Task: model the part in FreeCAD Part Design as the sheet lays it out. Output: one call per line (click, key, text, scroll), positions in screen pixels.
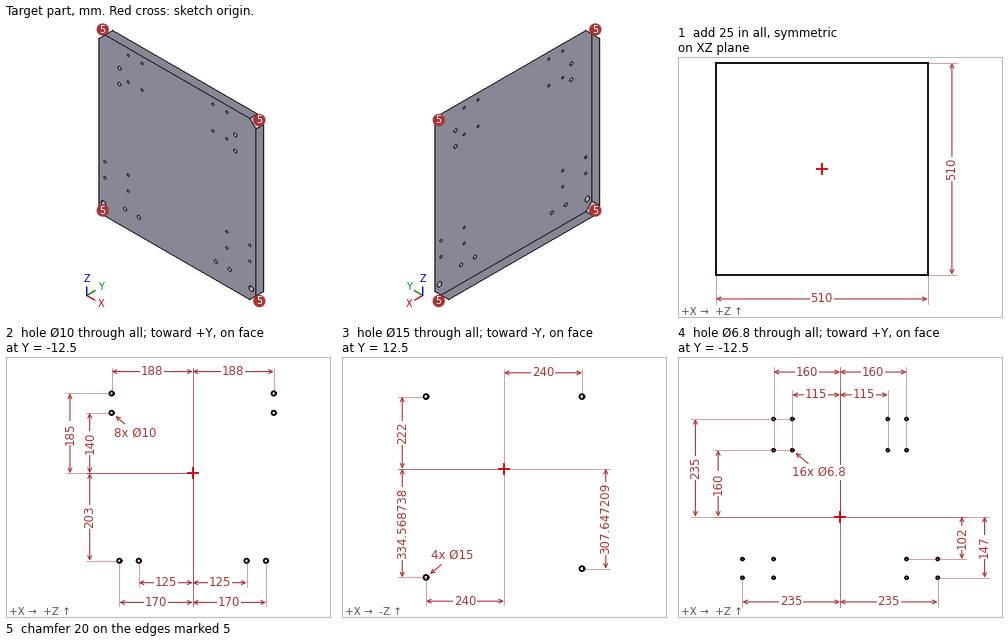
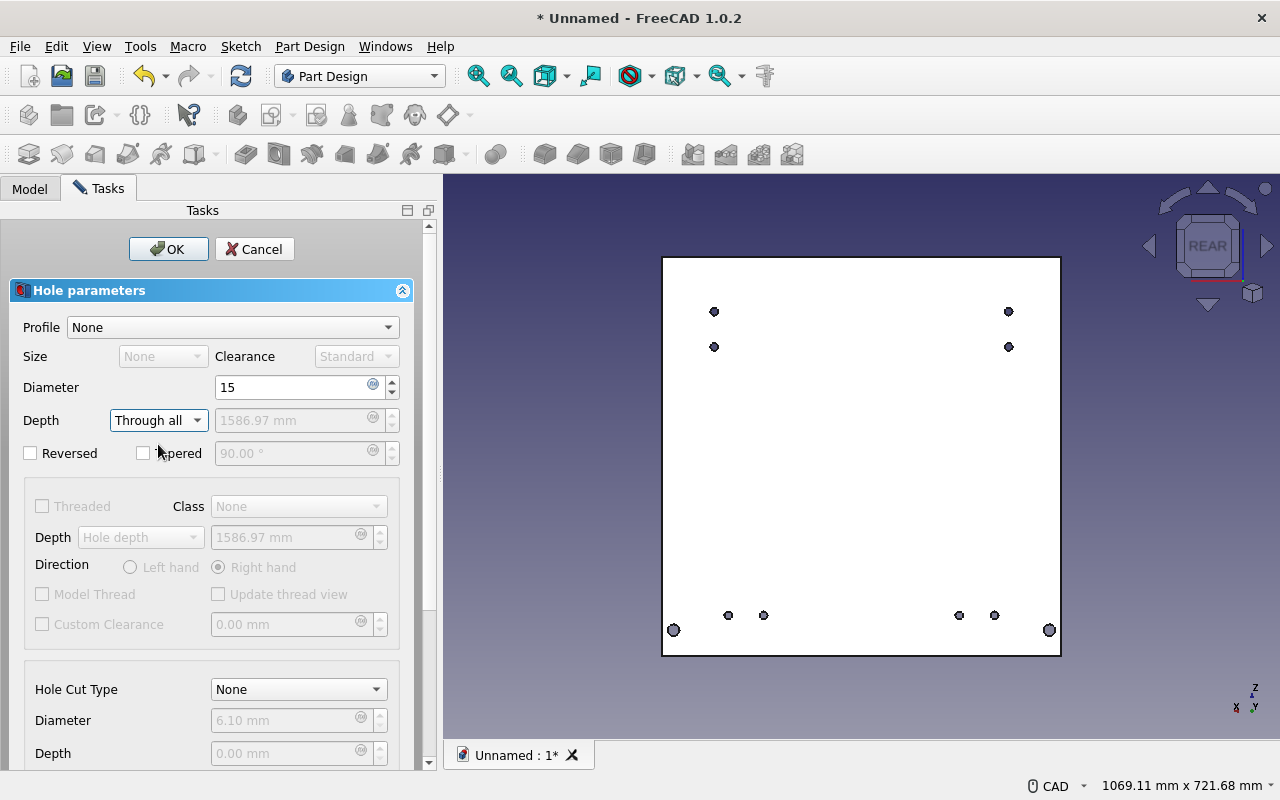
click(169, 249)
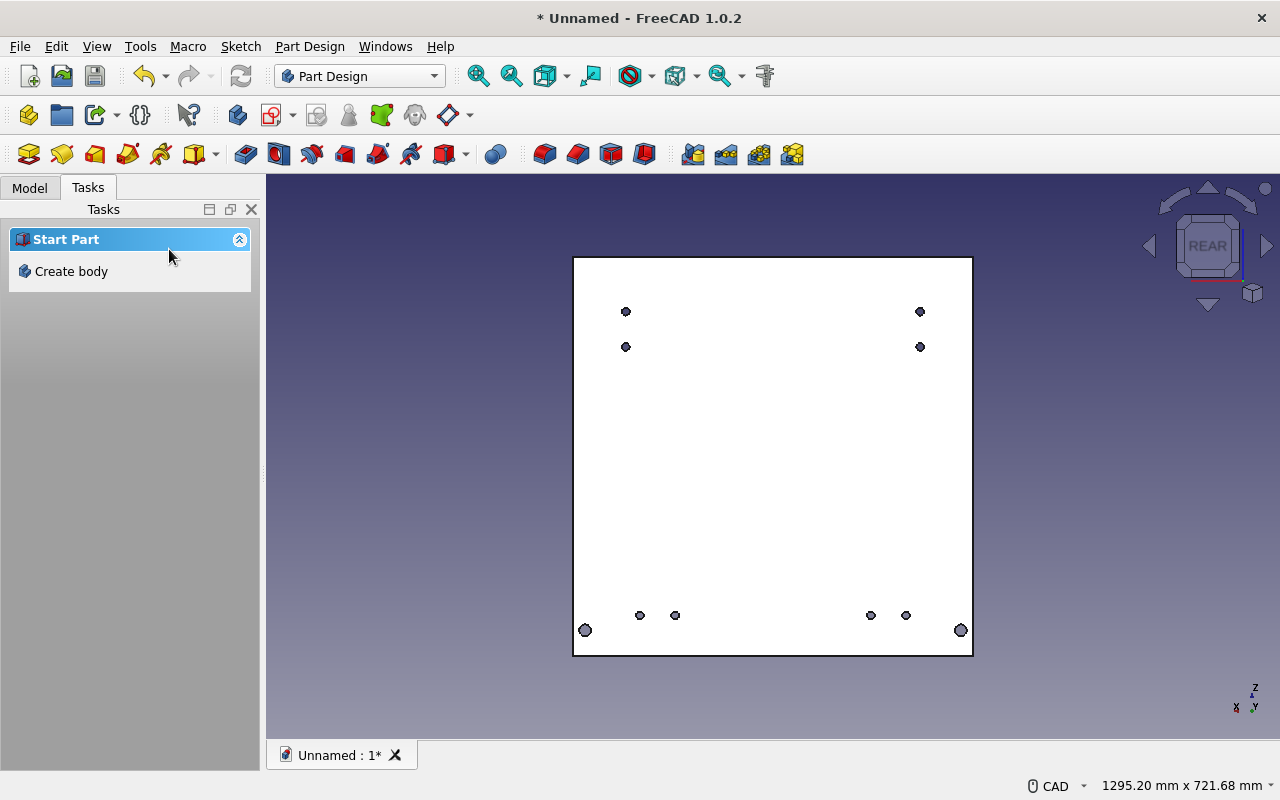
key(0)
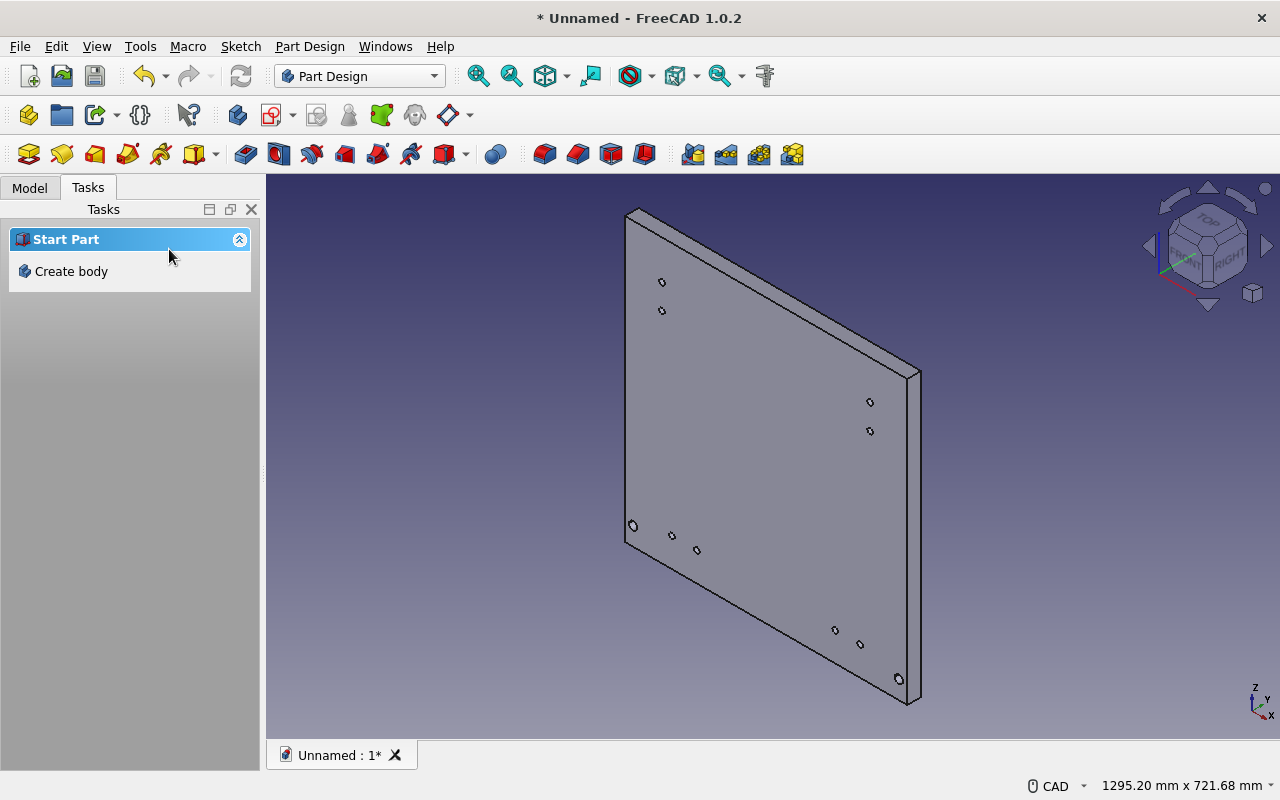
click(766, 459)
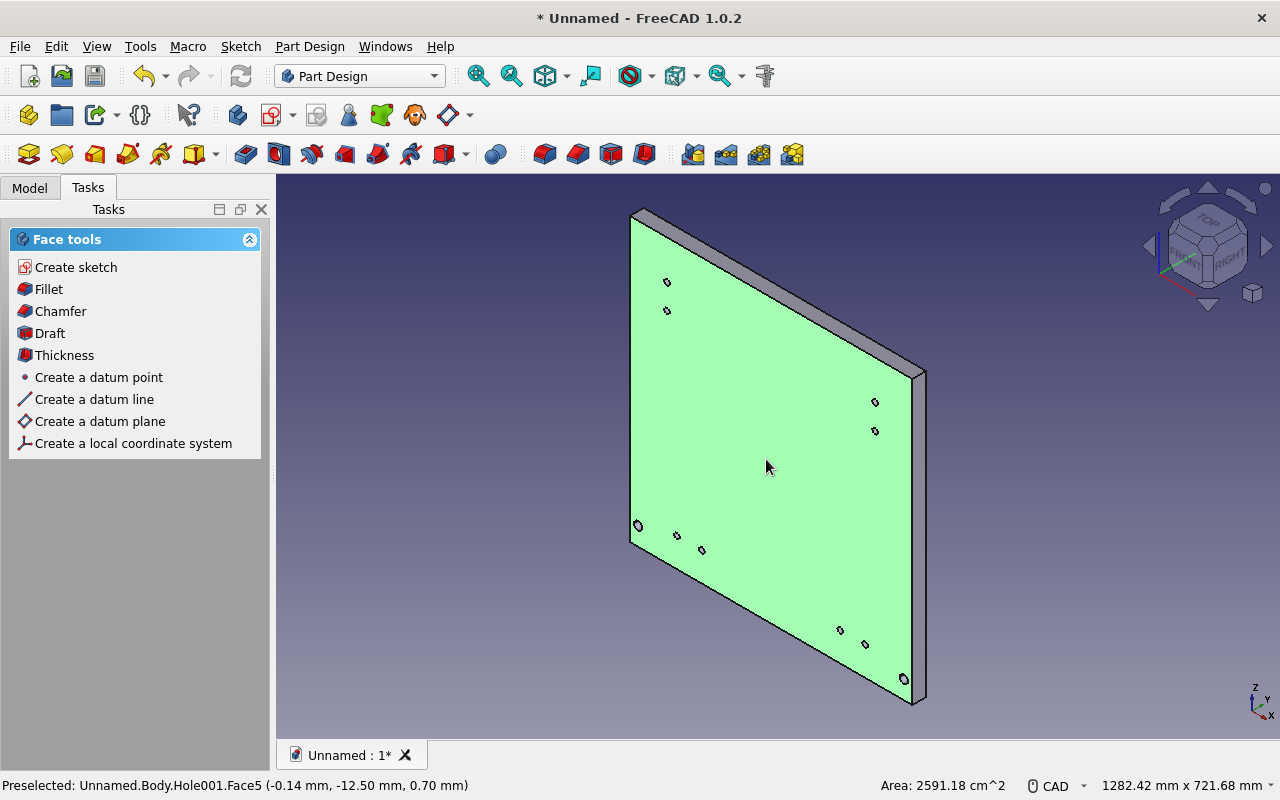
click(270, 116)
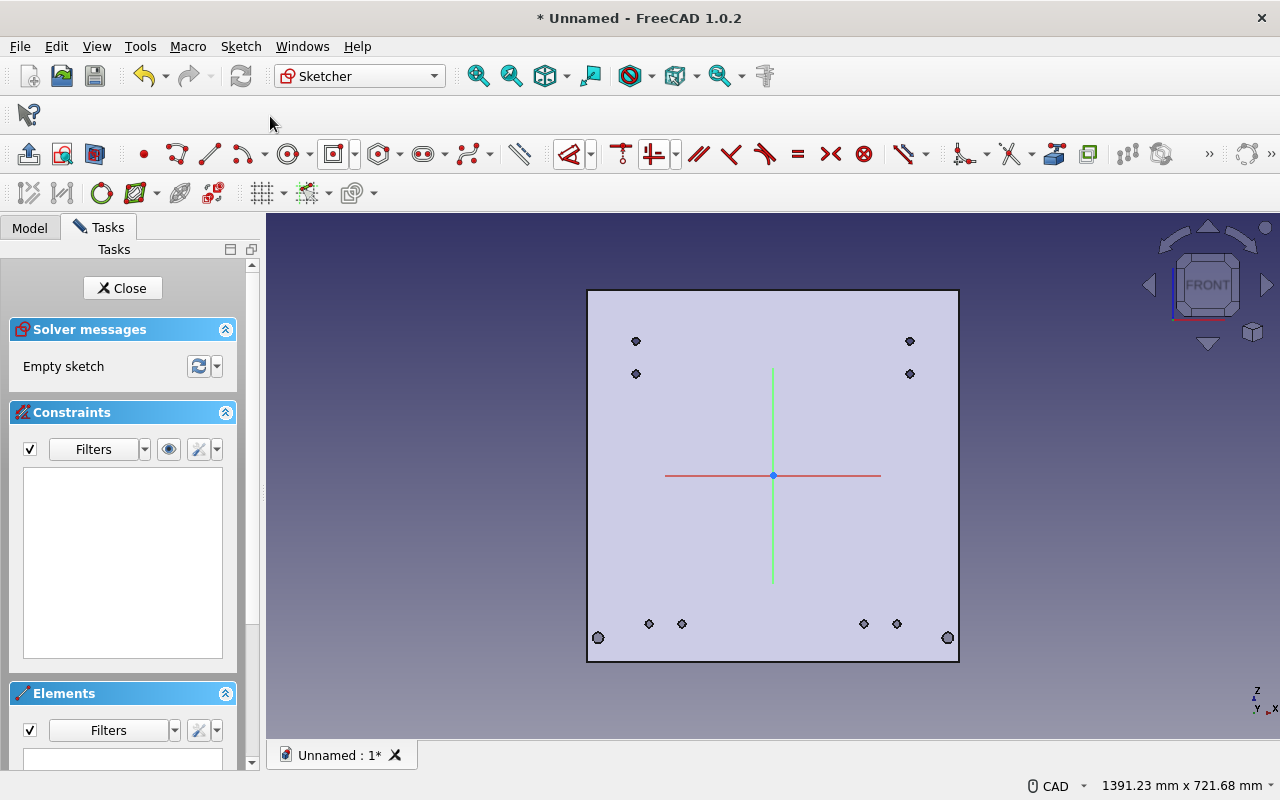
key(g)
key(c)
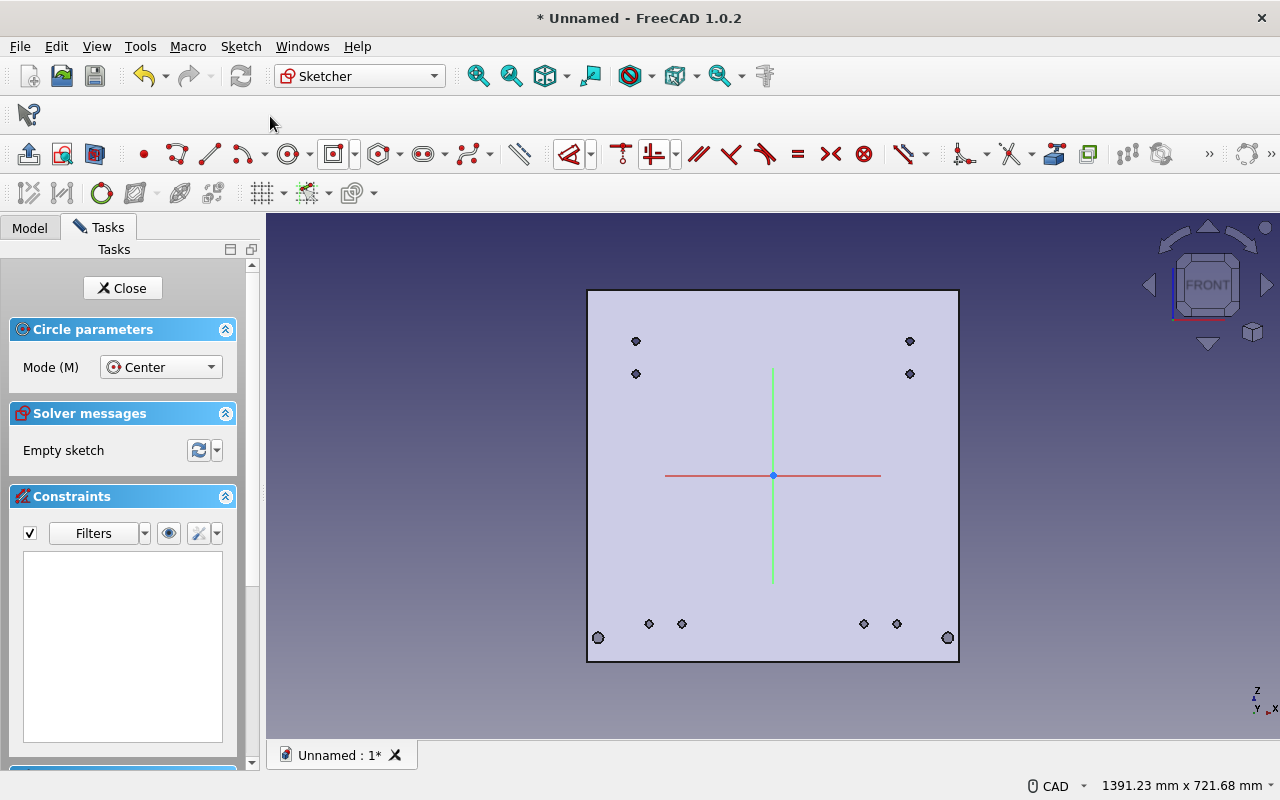
scroll(689, 359, up, 12)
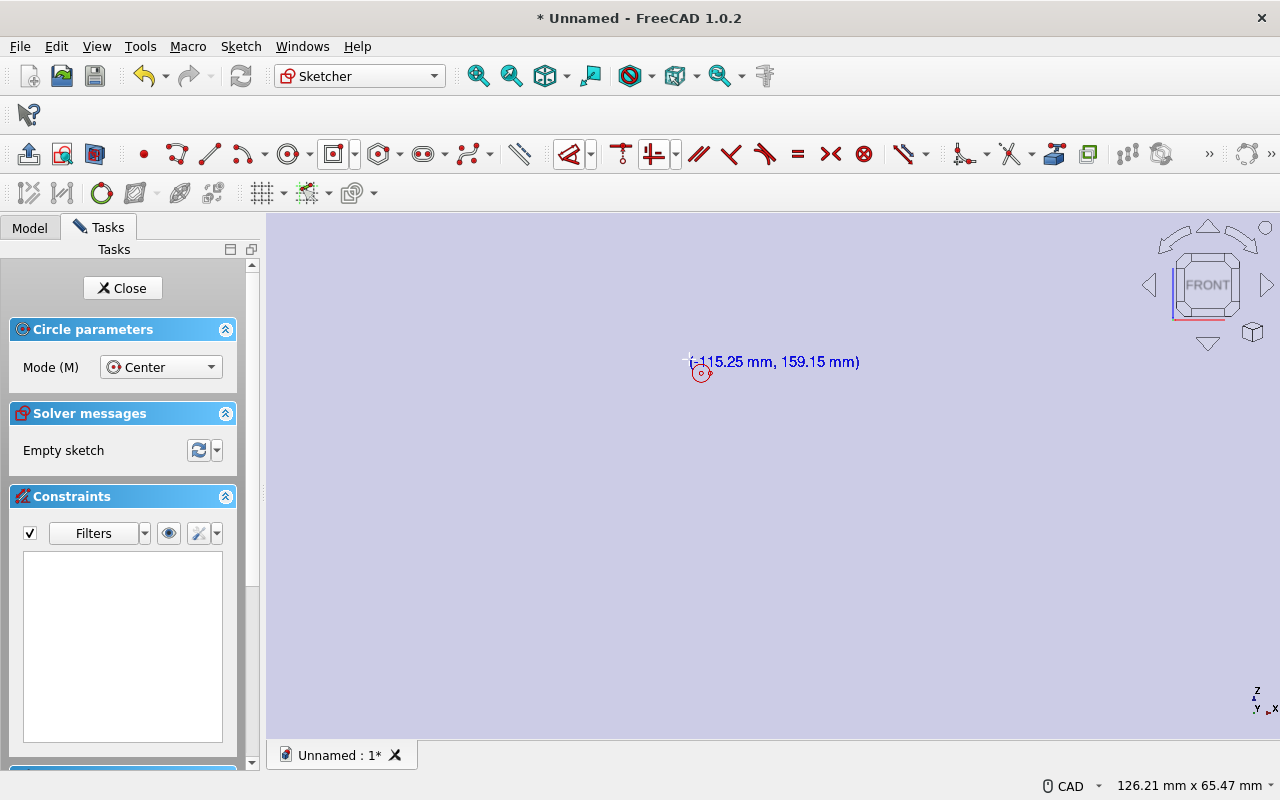
scroll(592, 374, down, 11)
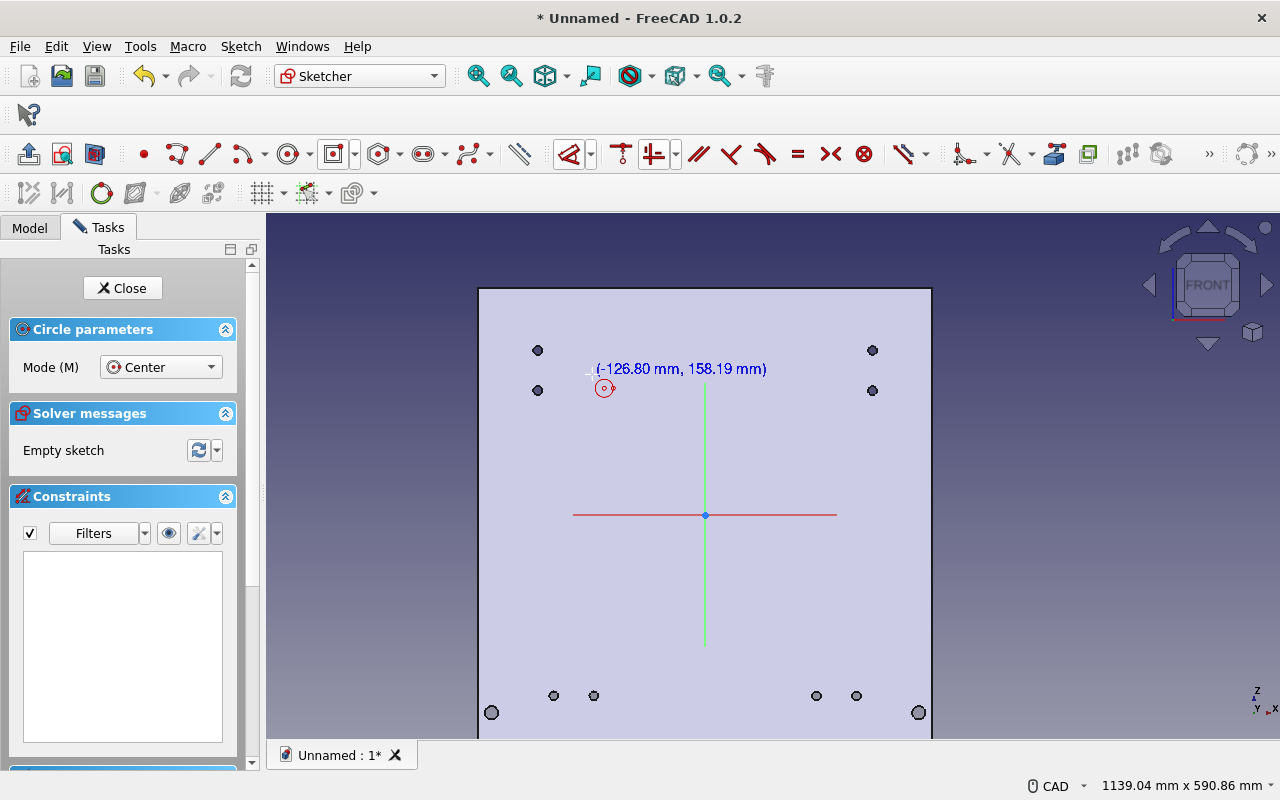
click(603, 373)
move(605, 371)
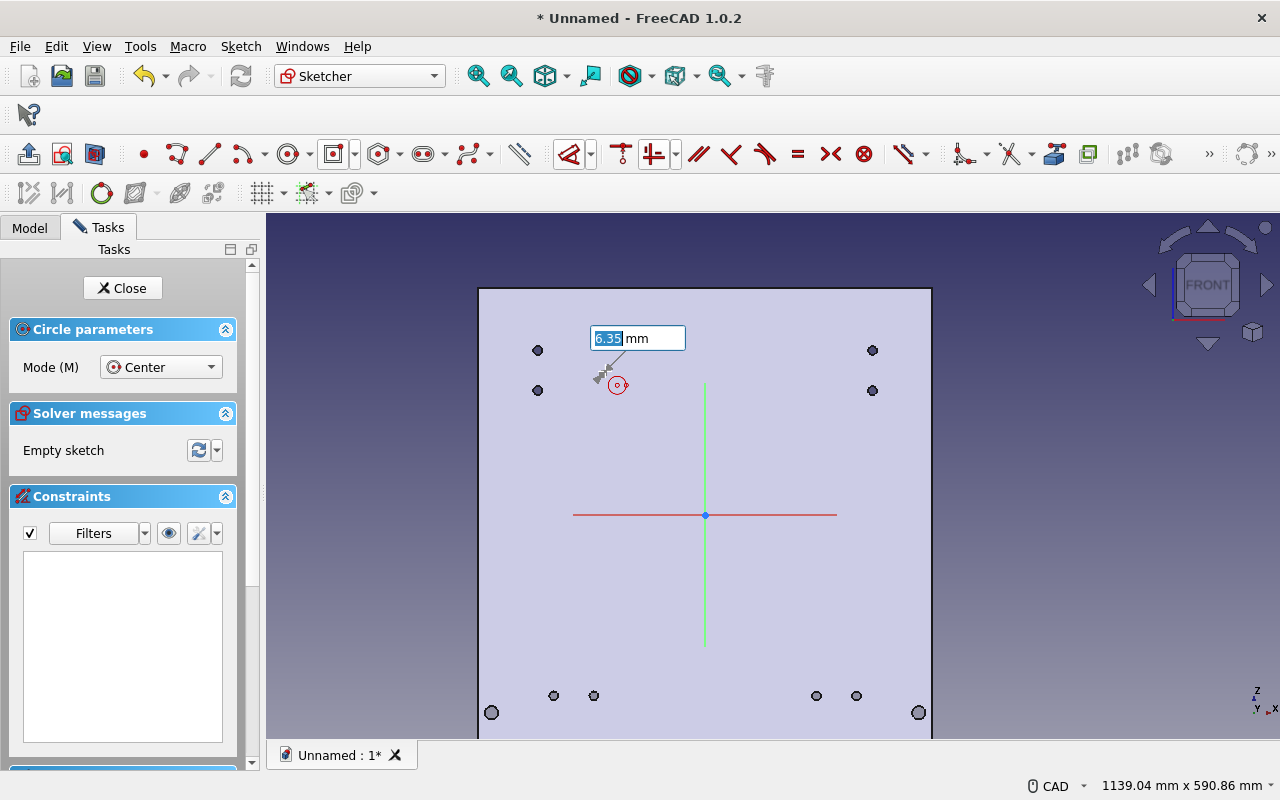
text(6.8)
key(Return)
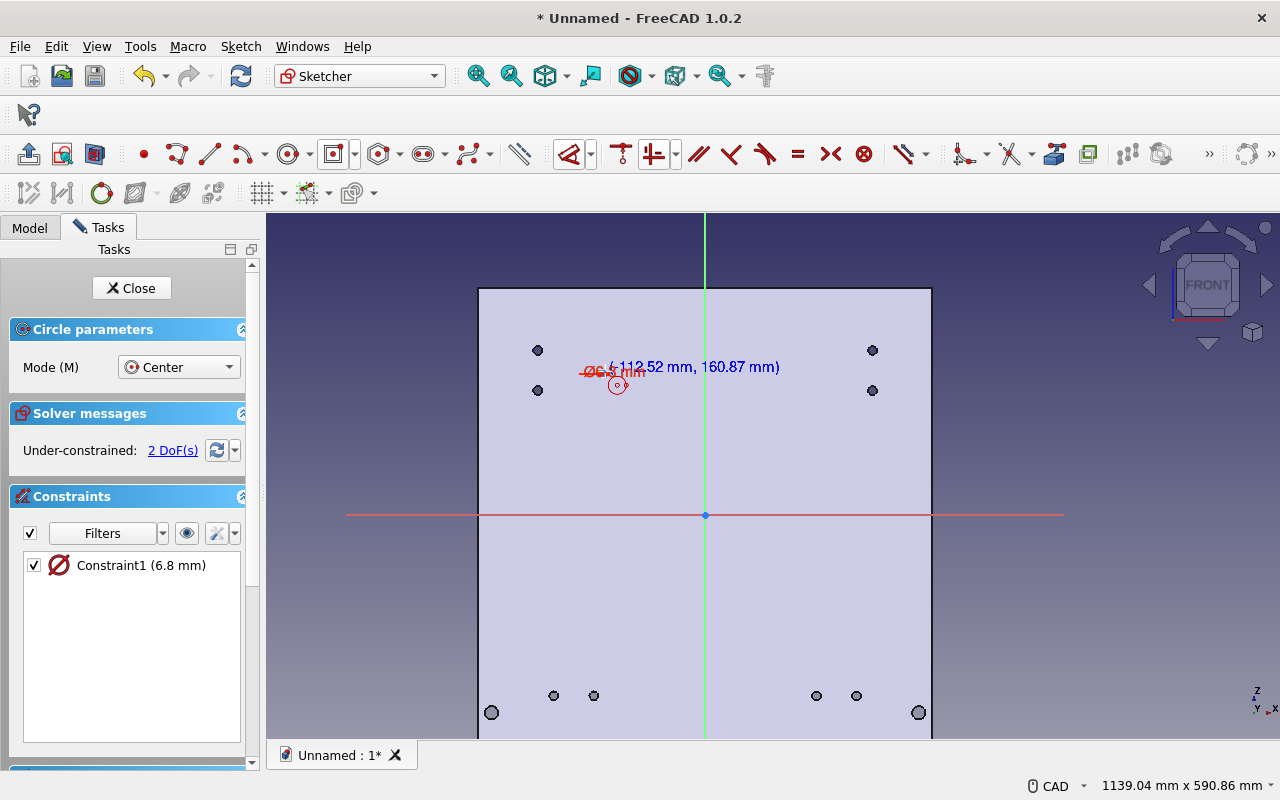
scroll(563, 373, up, 11)